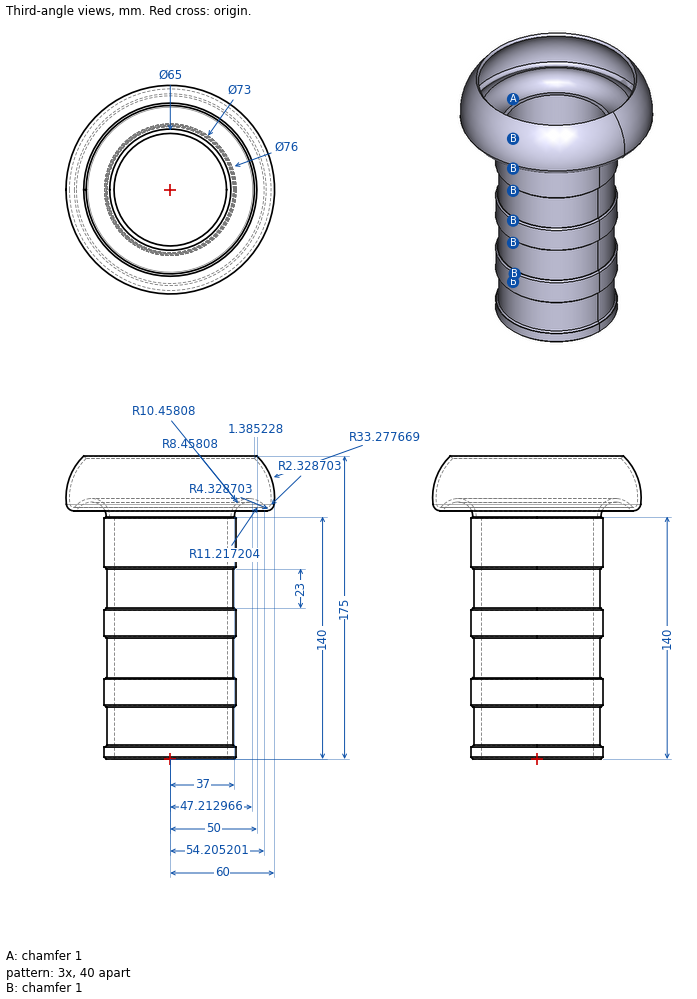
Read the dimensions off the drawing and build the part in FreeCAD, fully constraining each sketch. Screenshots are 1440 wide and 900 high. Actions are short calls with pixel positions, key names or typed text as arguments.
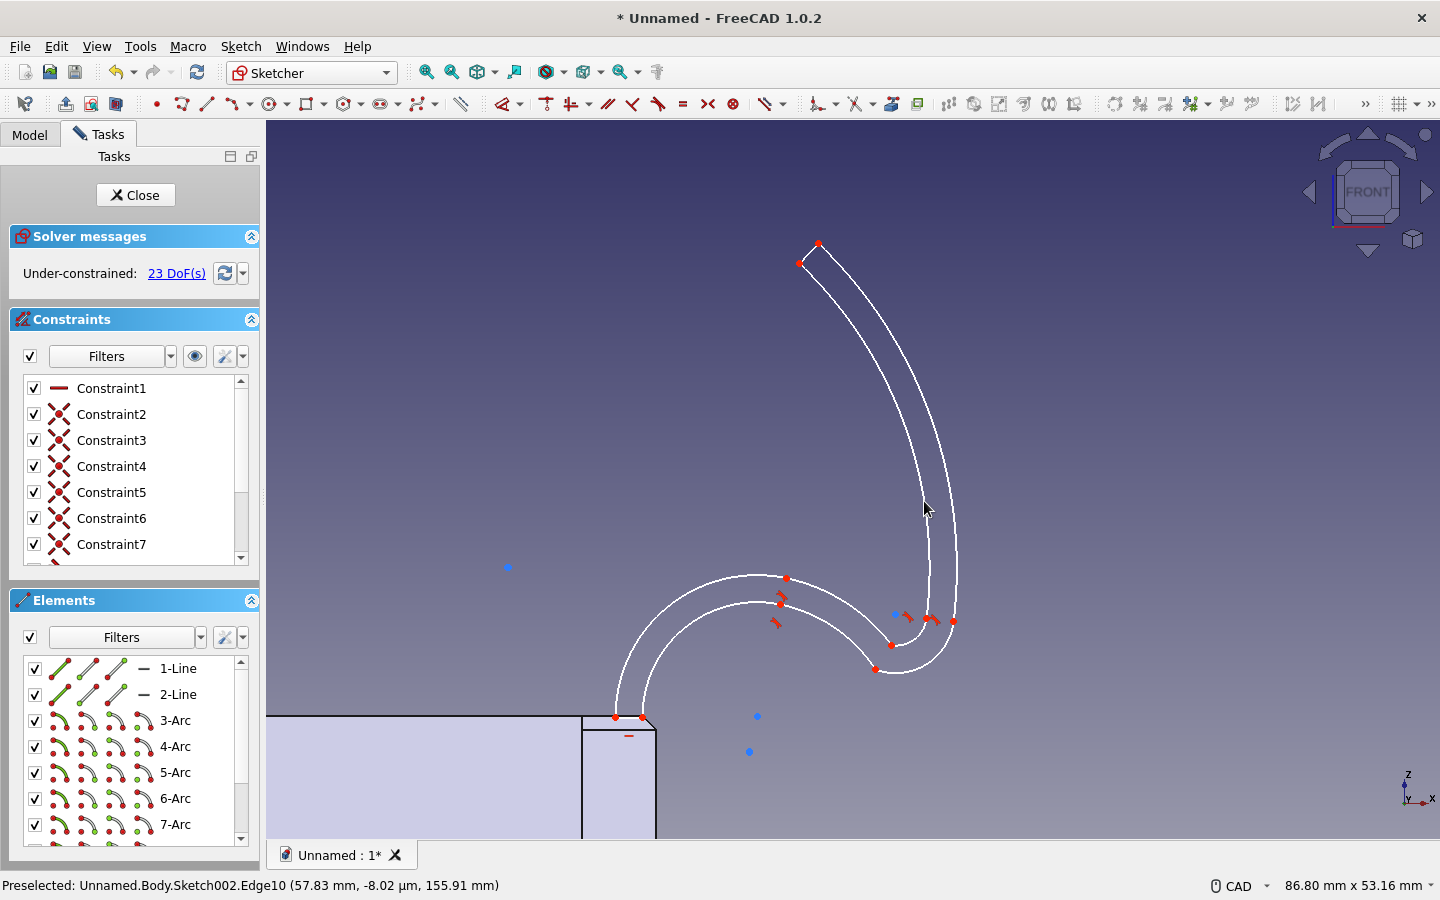
click(720, 608)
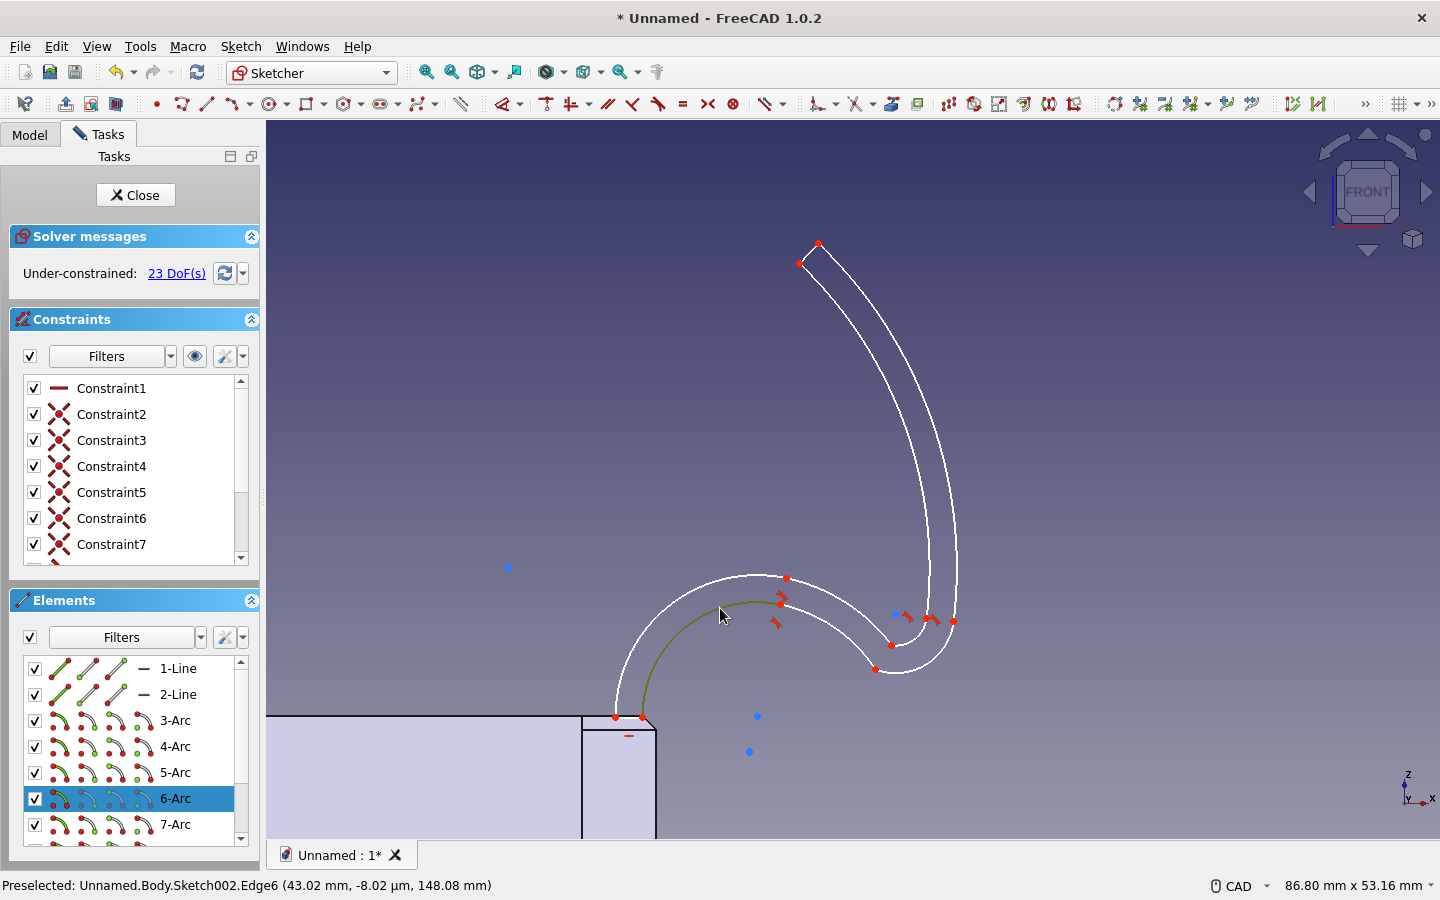
click(712, 583)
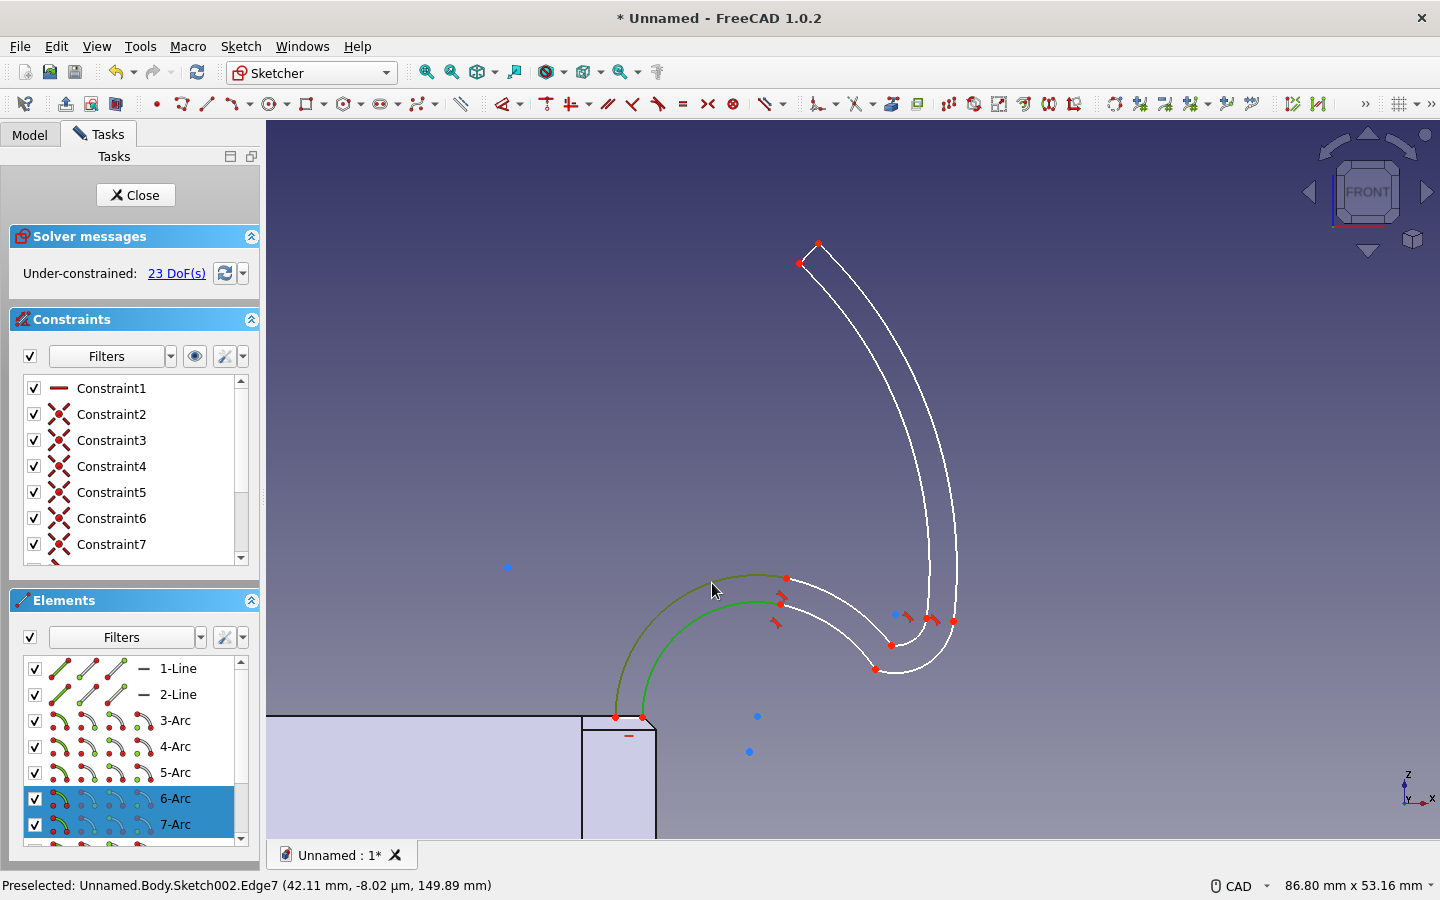
click(546, 104)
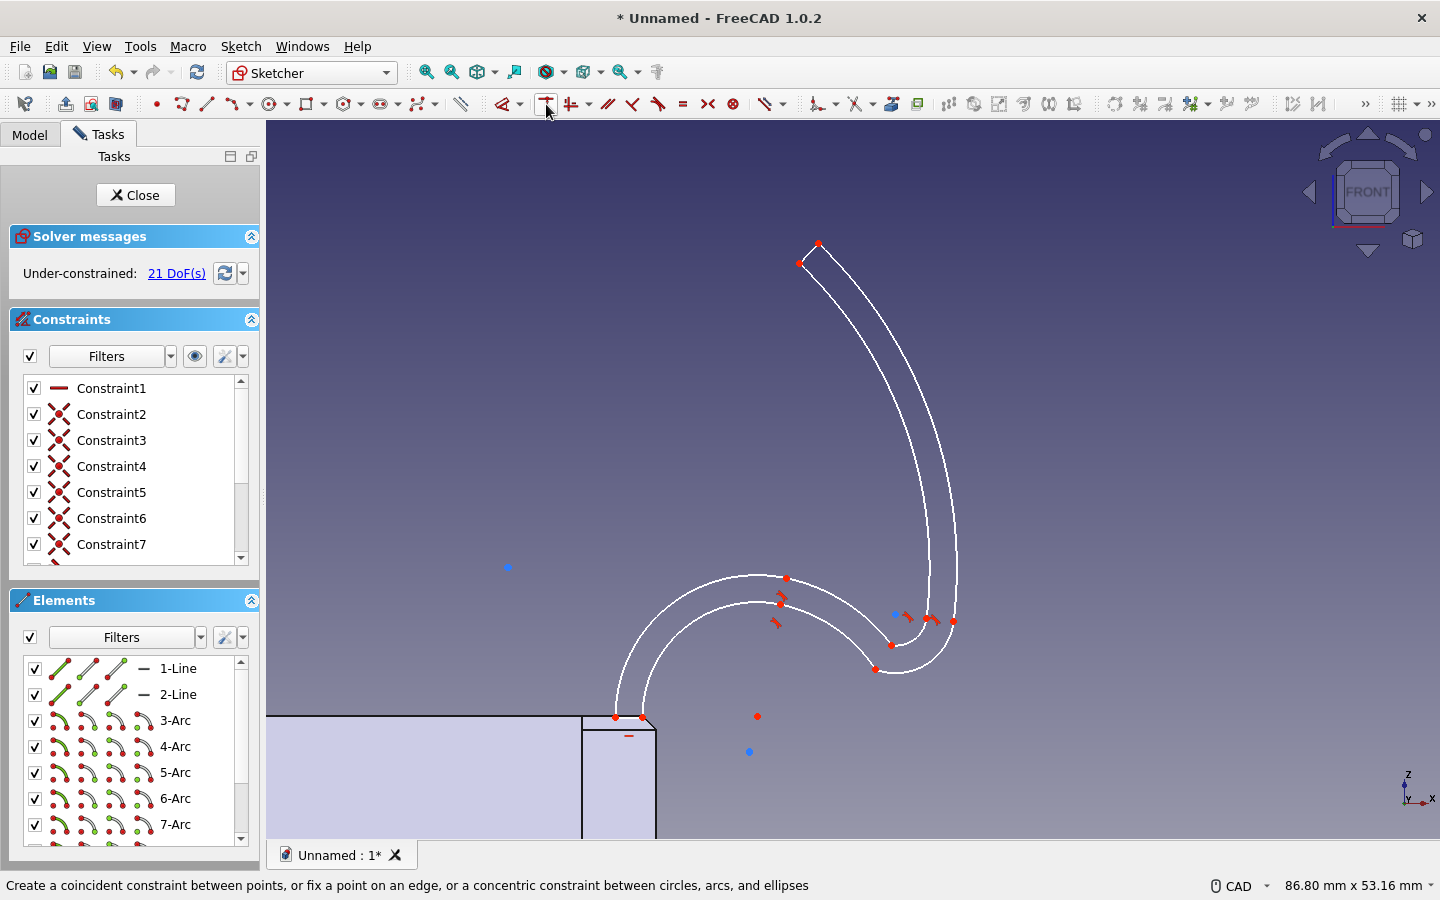
click(853, 642)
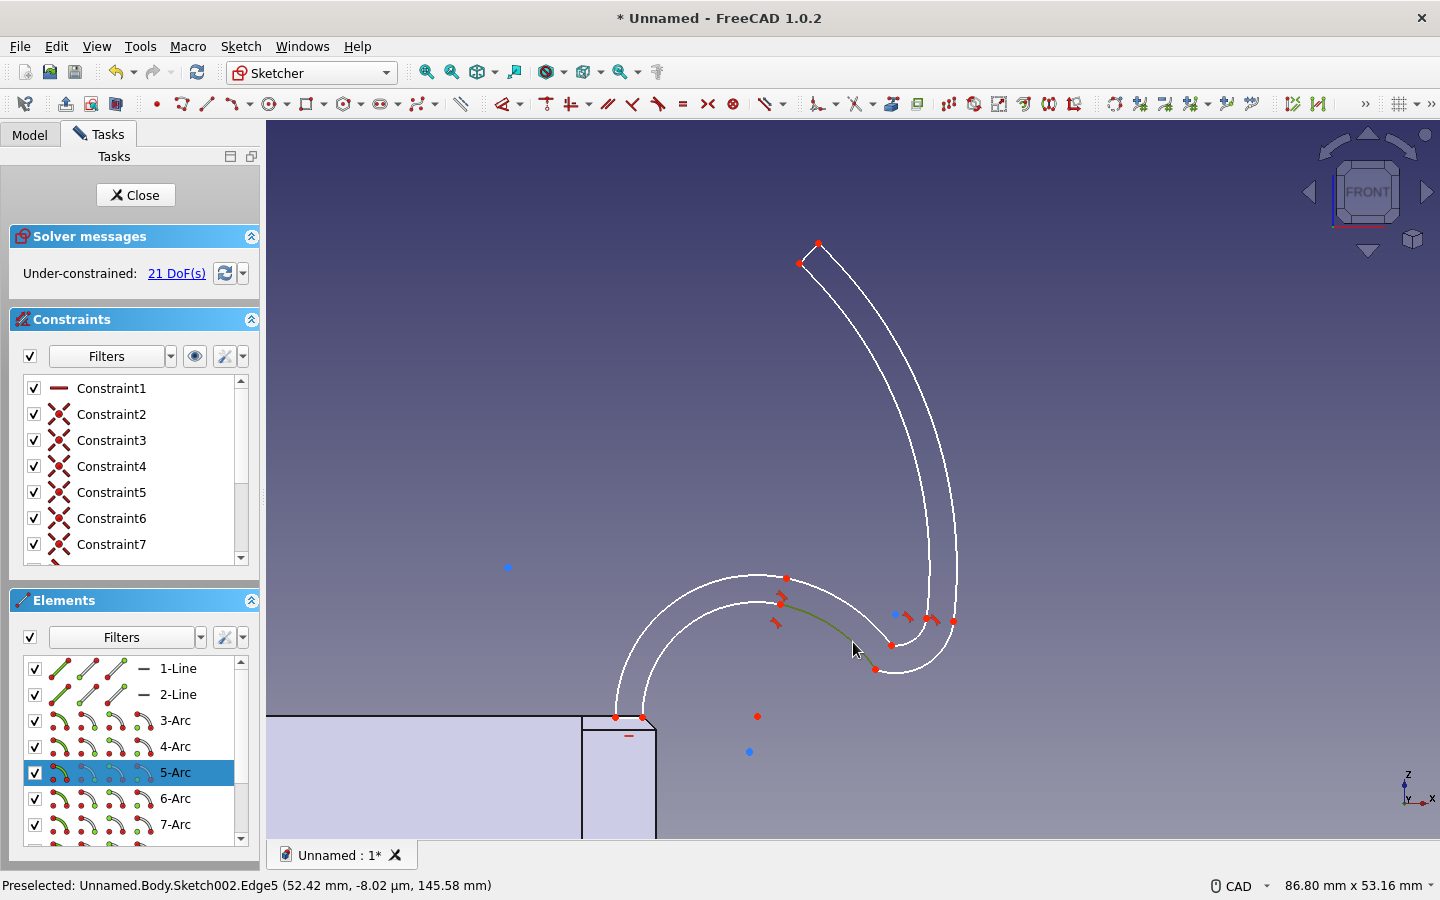
click(866, 617)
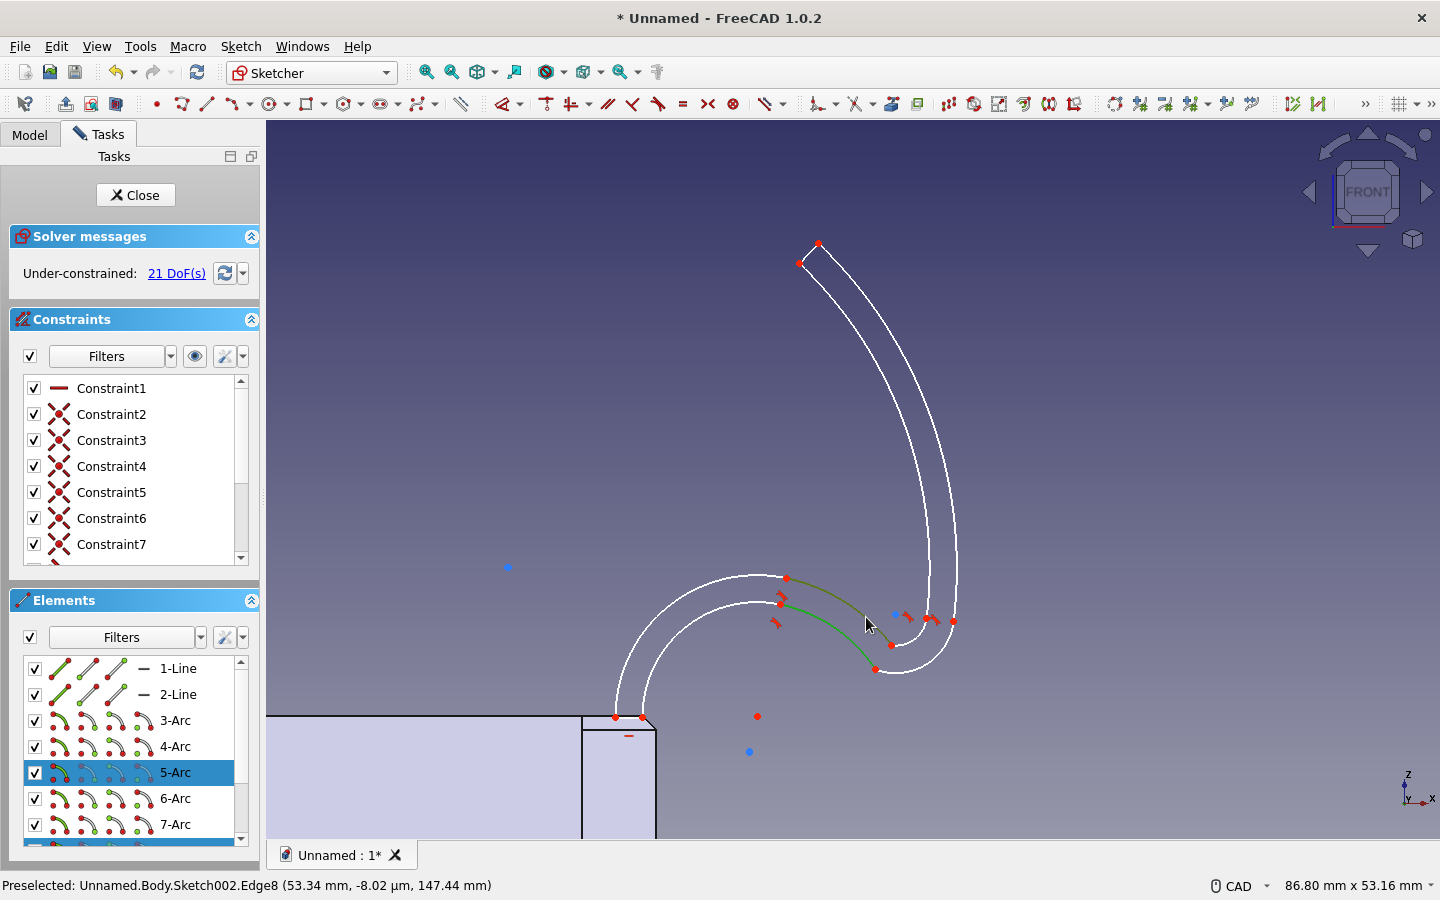
click(546, 104)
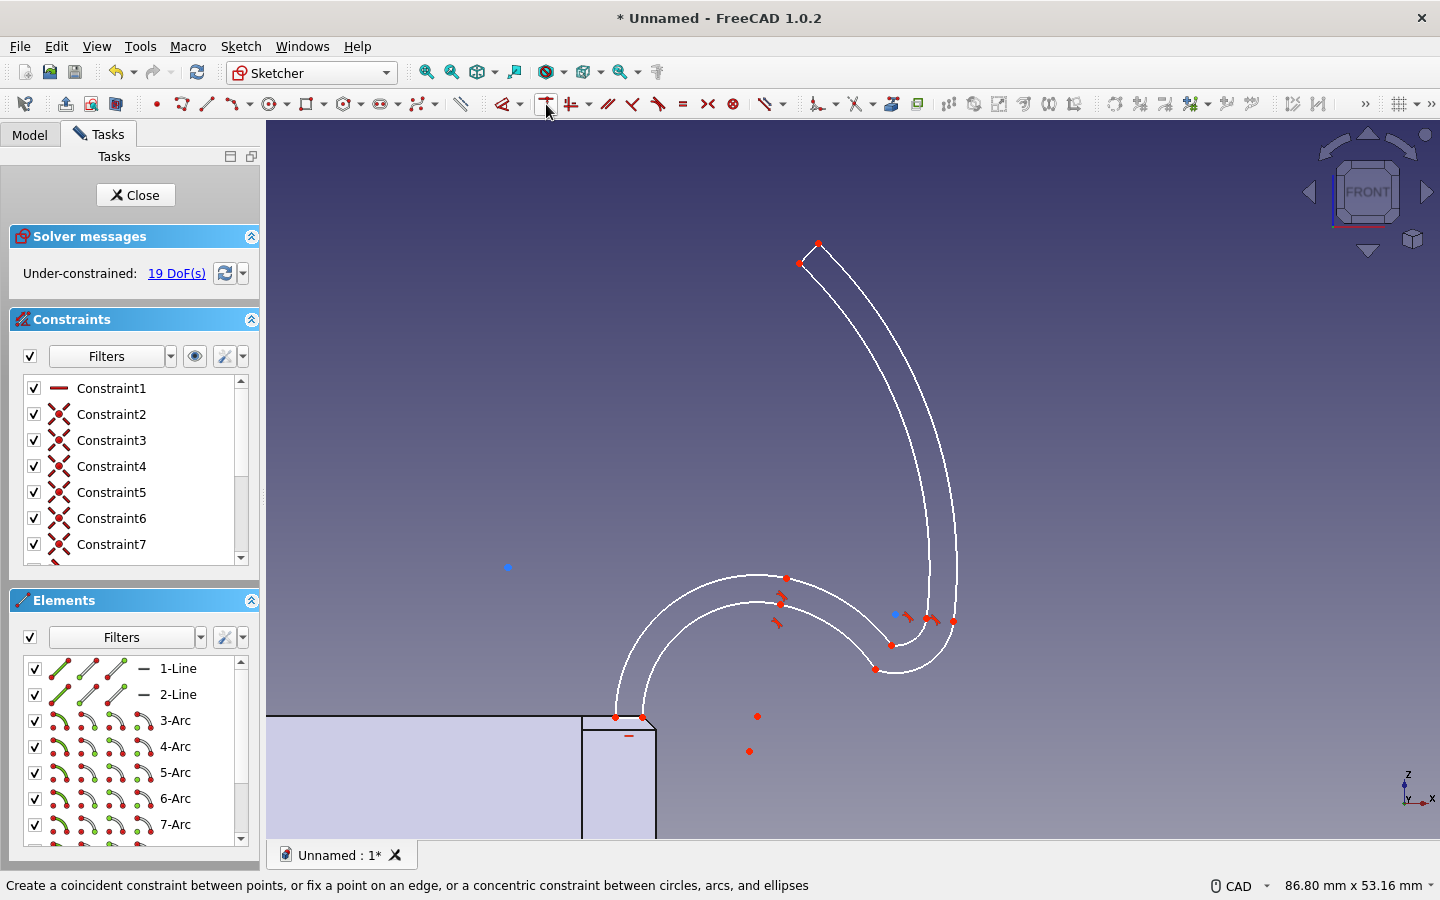
click(907, 672)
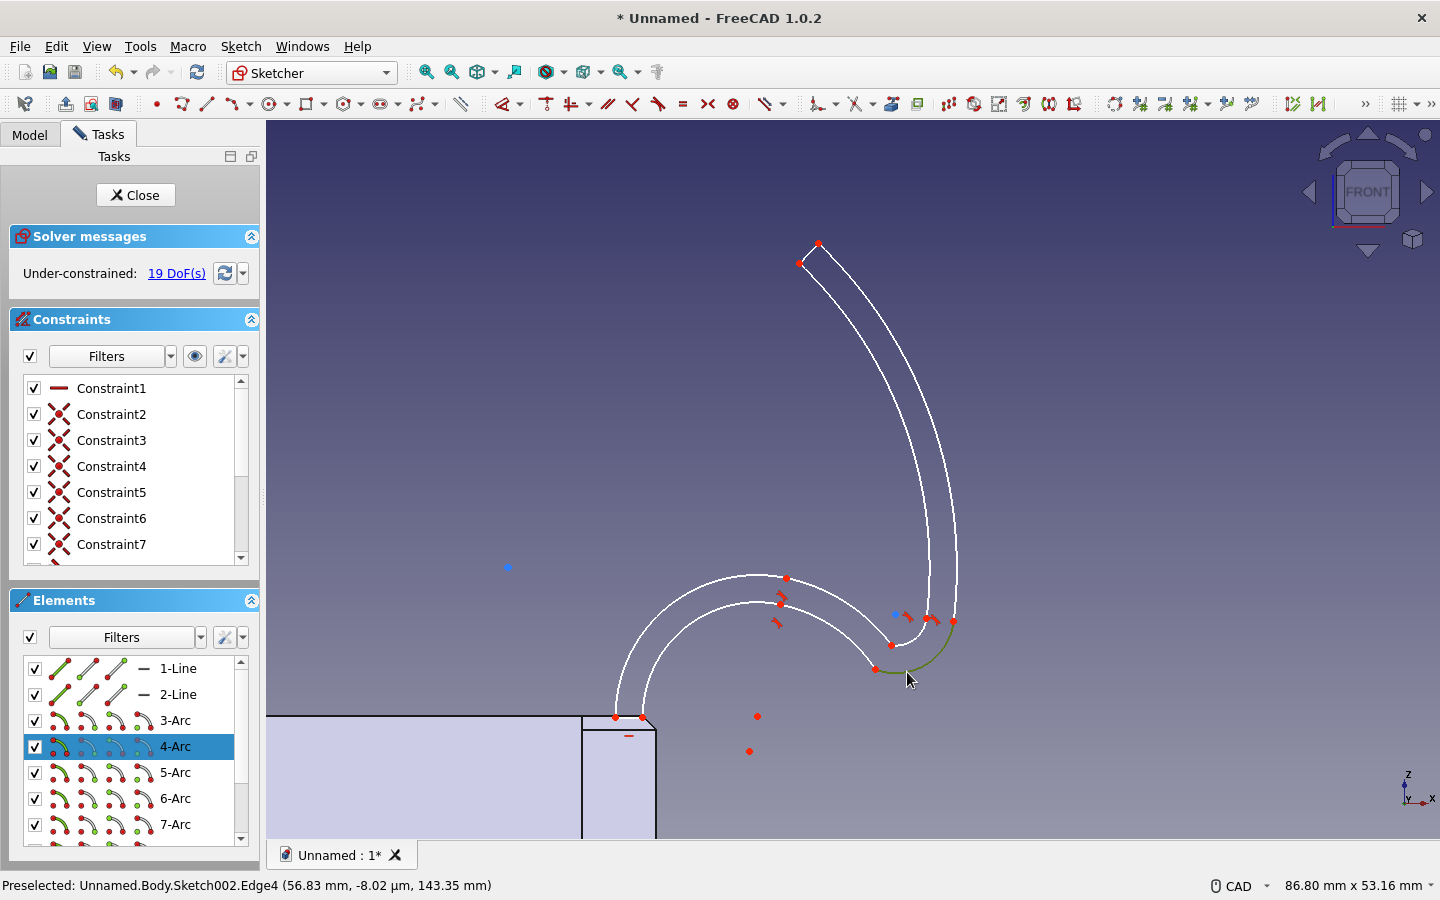
click(906, 644)